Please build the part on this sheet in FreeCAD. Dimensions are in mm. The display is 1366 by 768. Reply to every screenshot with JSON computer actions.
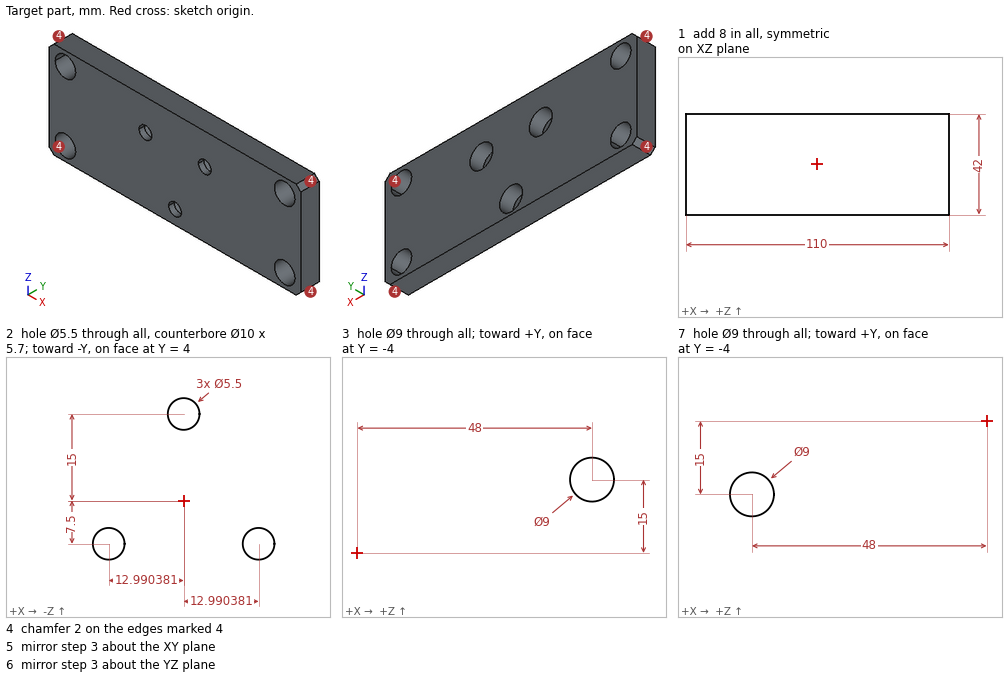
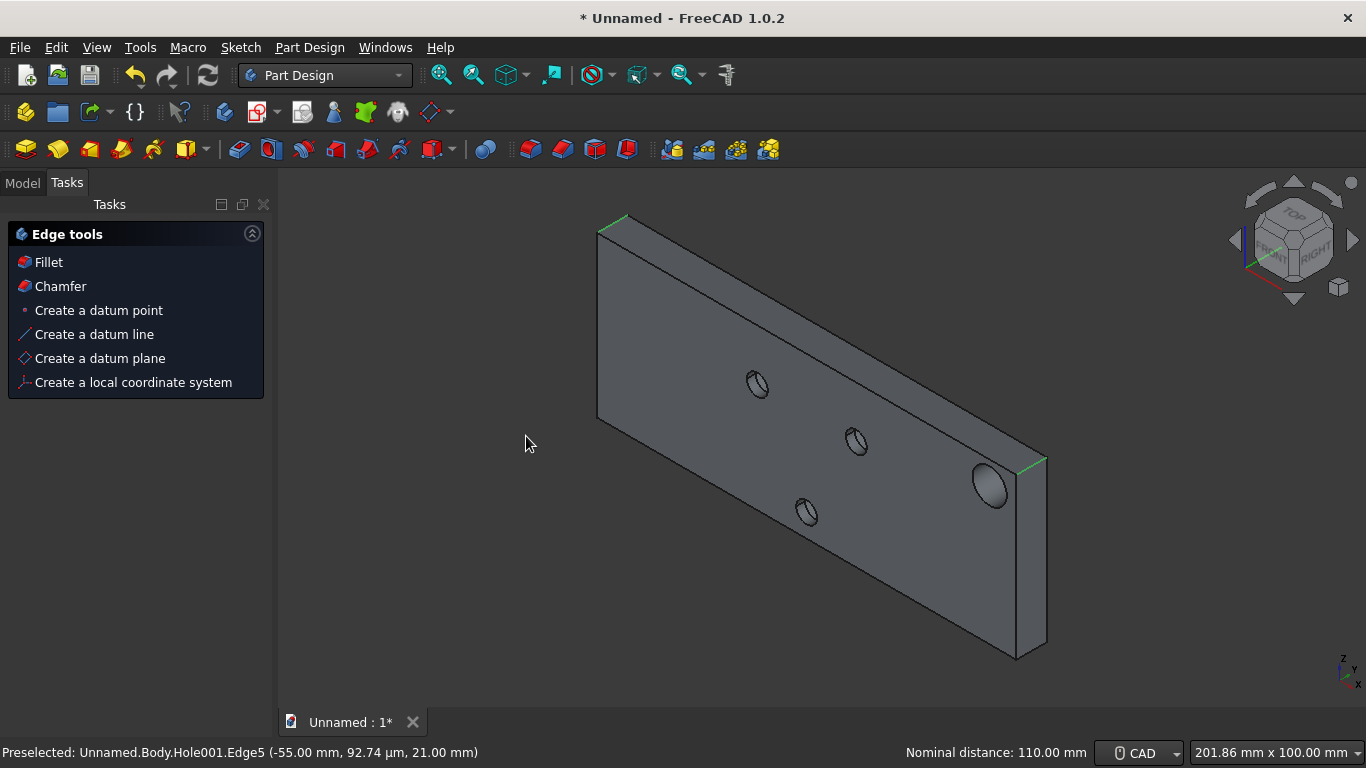
{"action": "key", "text": "1"}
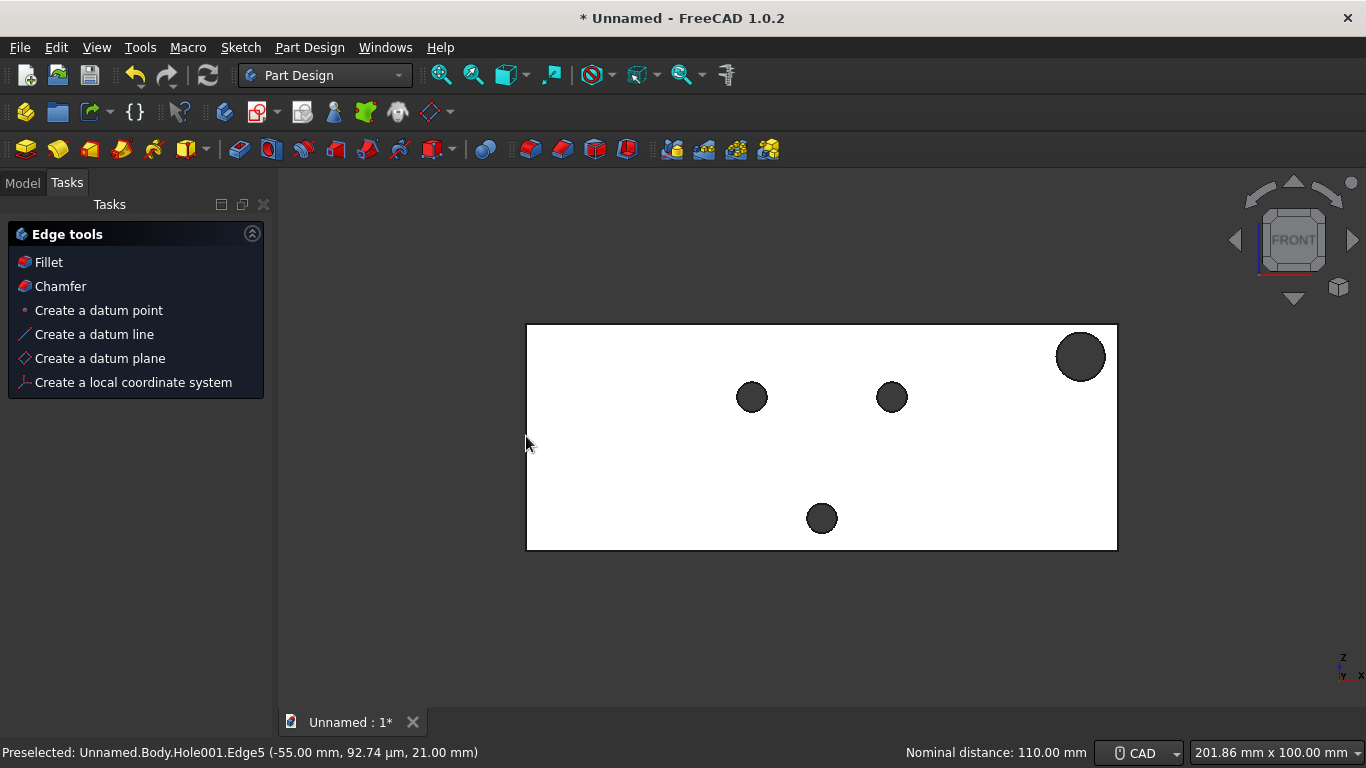
{"action": "key", "text": "3"}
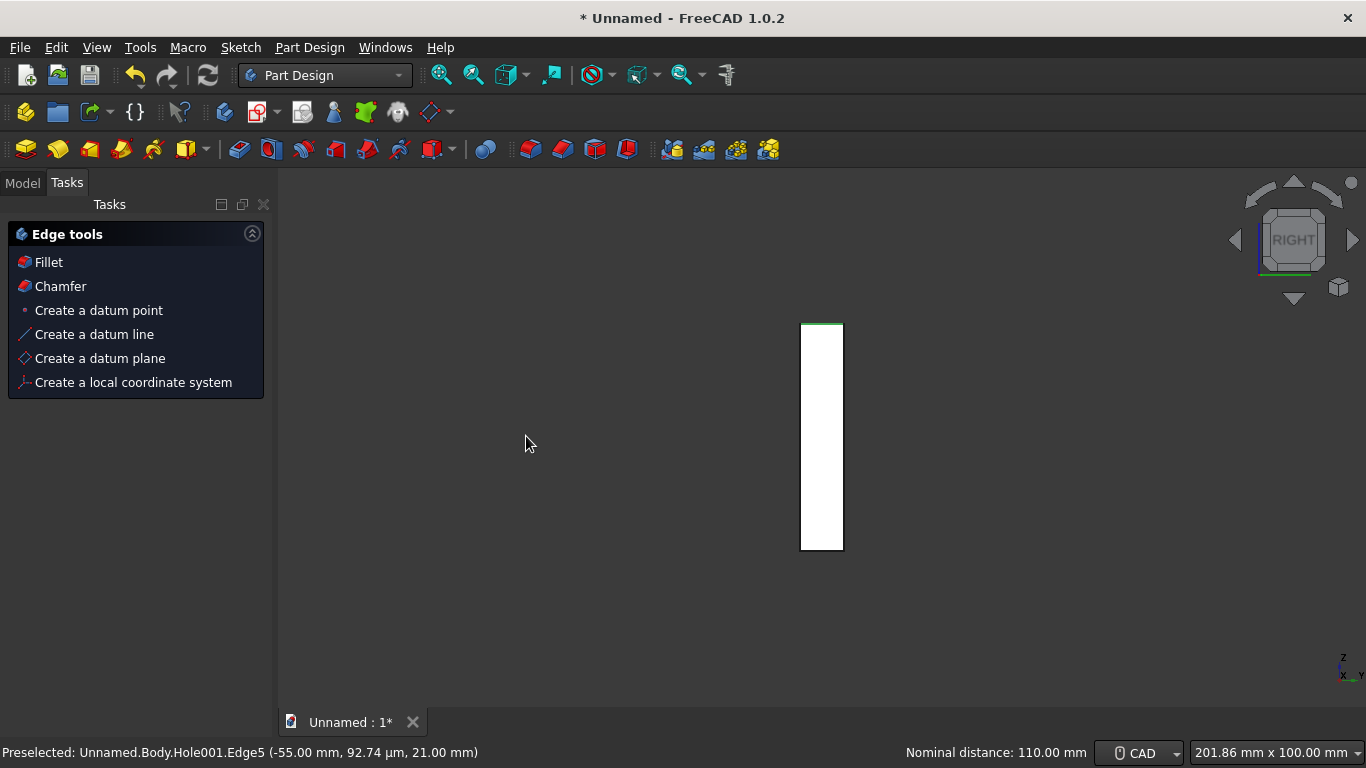
{"action": "left_click", "coordinate": [442, 76]}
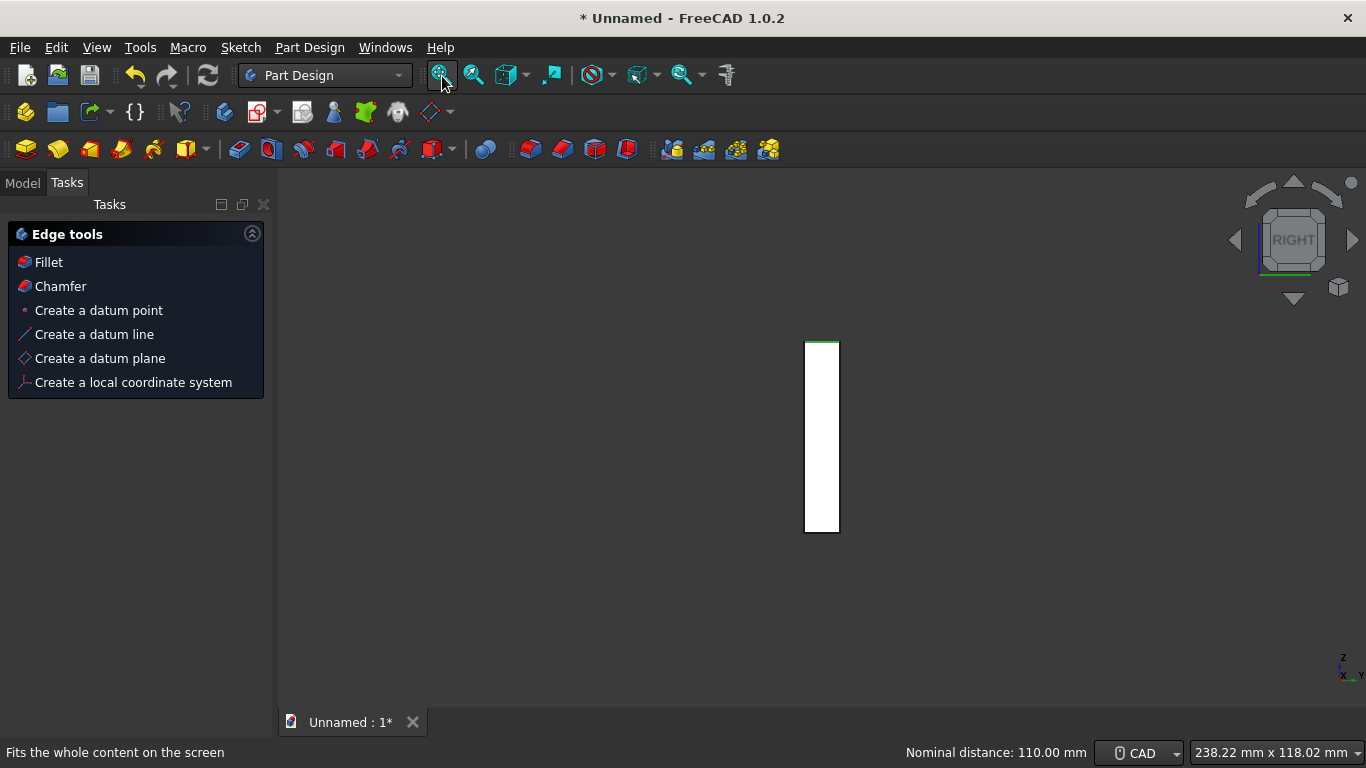
{"action": "left_click", "coordinate": [822, 532], "text": "ctrl"}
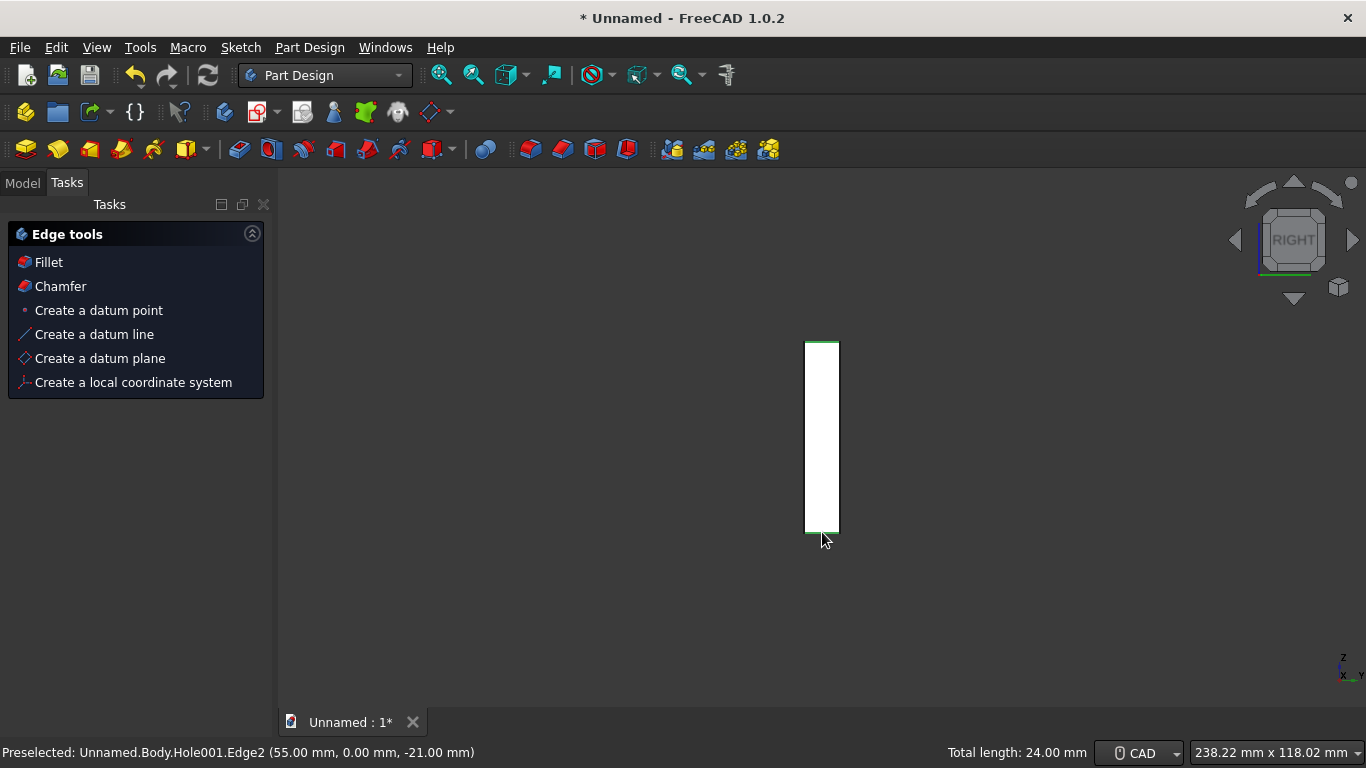
{"action": "key", "text": "5"}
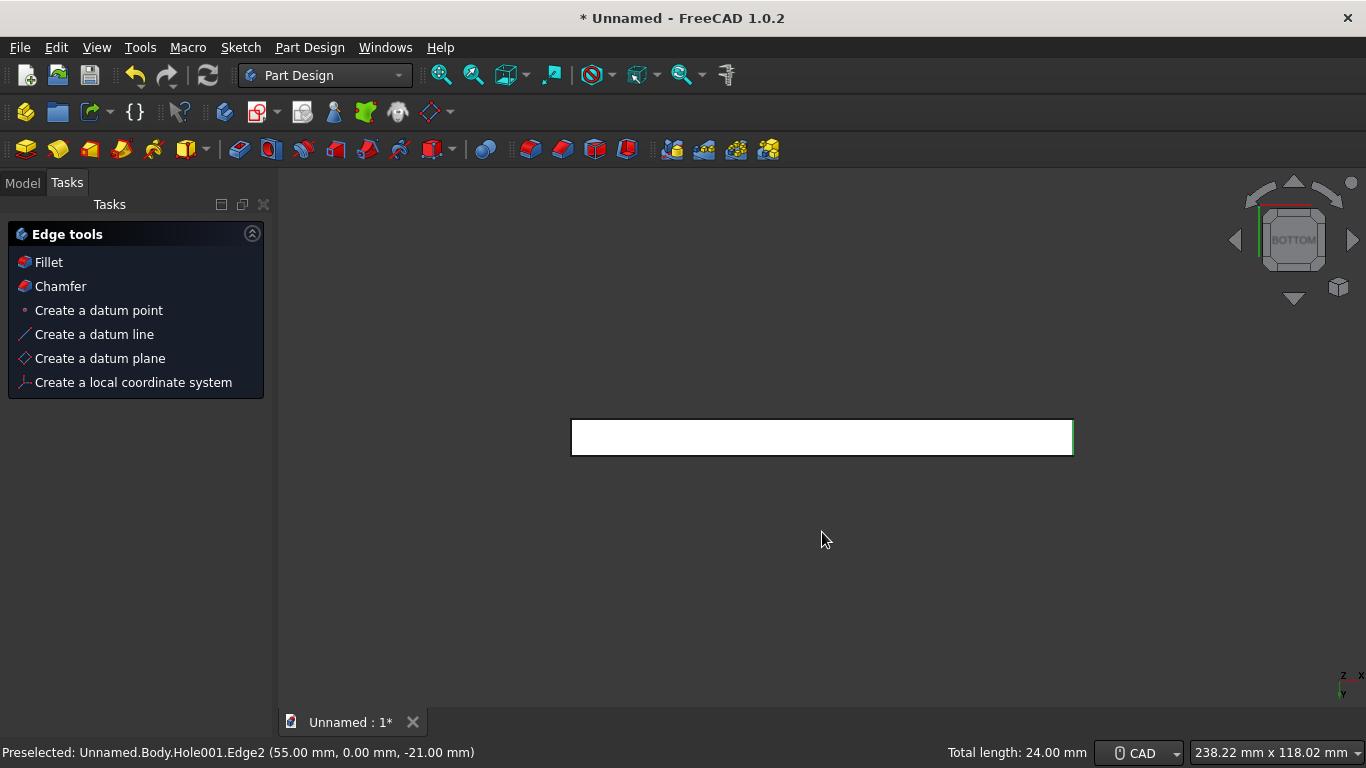
{"action": "left_click", "coordinate": [571, 436], "text": "ctrl"}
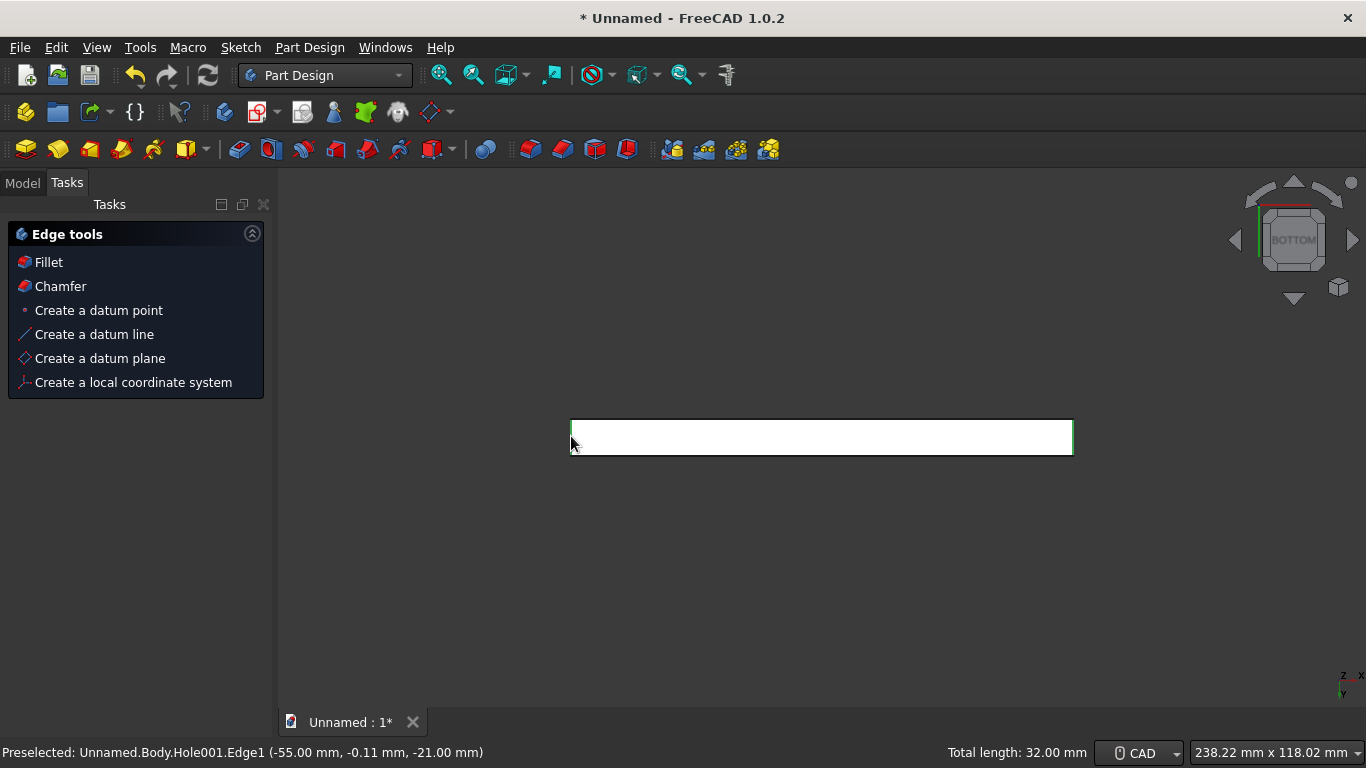
{"action": "left_click", "coordinate": [564, 150]}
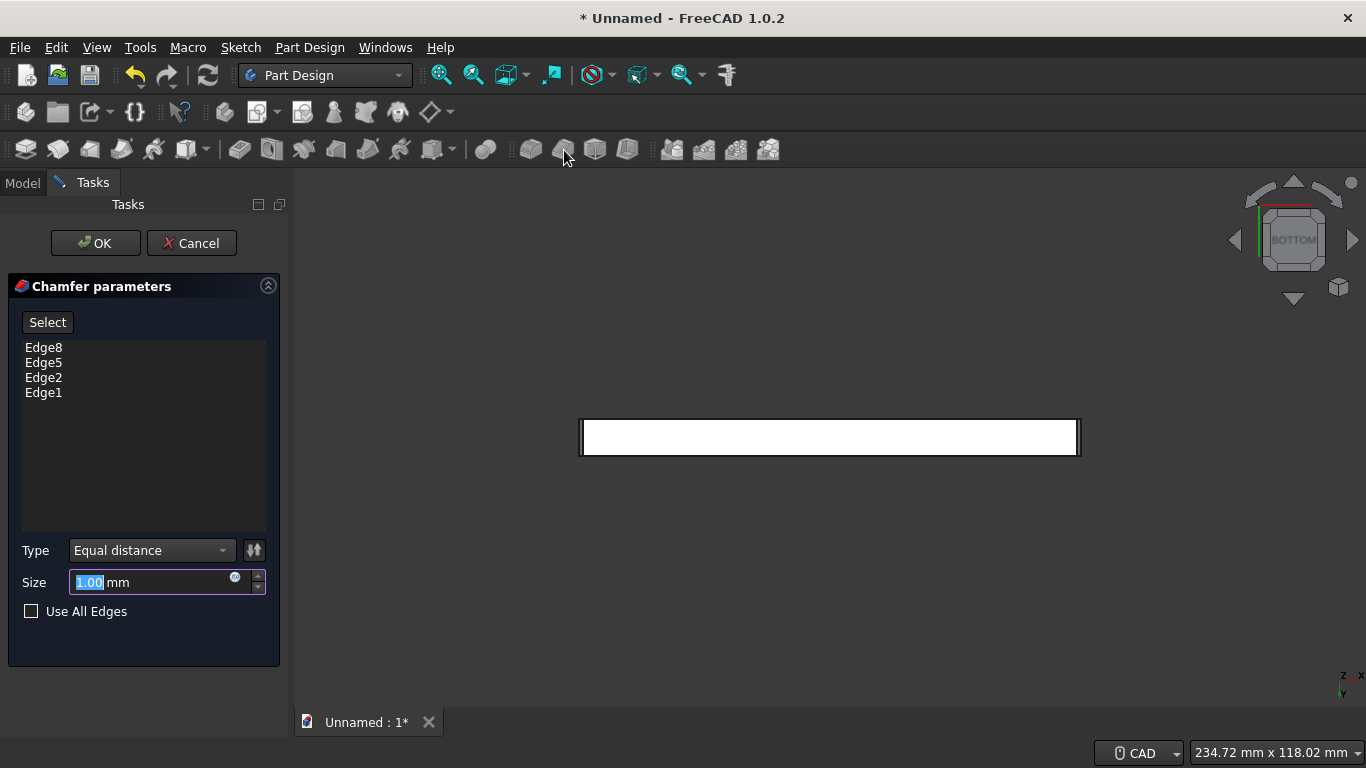
{"action": "type", "text": "2"}
{"action": "key", "text": "Tab"}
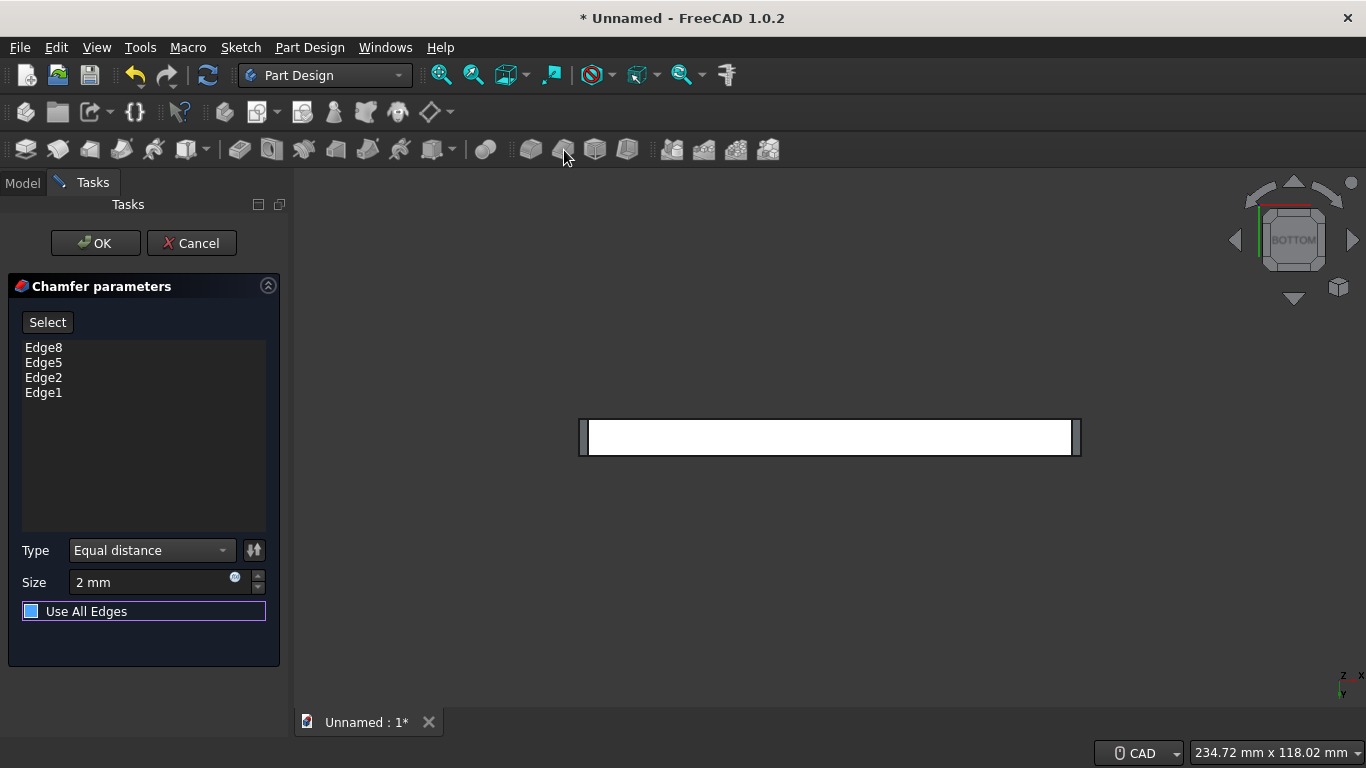
{"action": "left_click", "coordinate": [96, 243]}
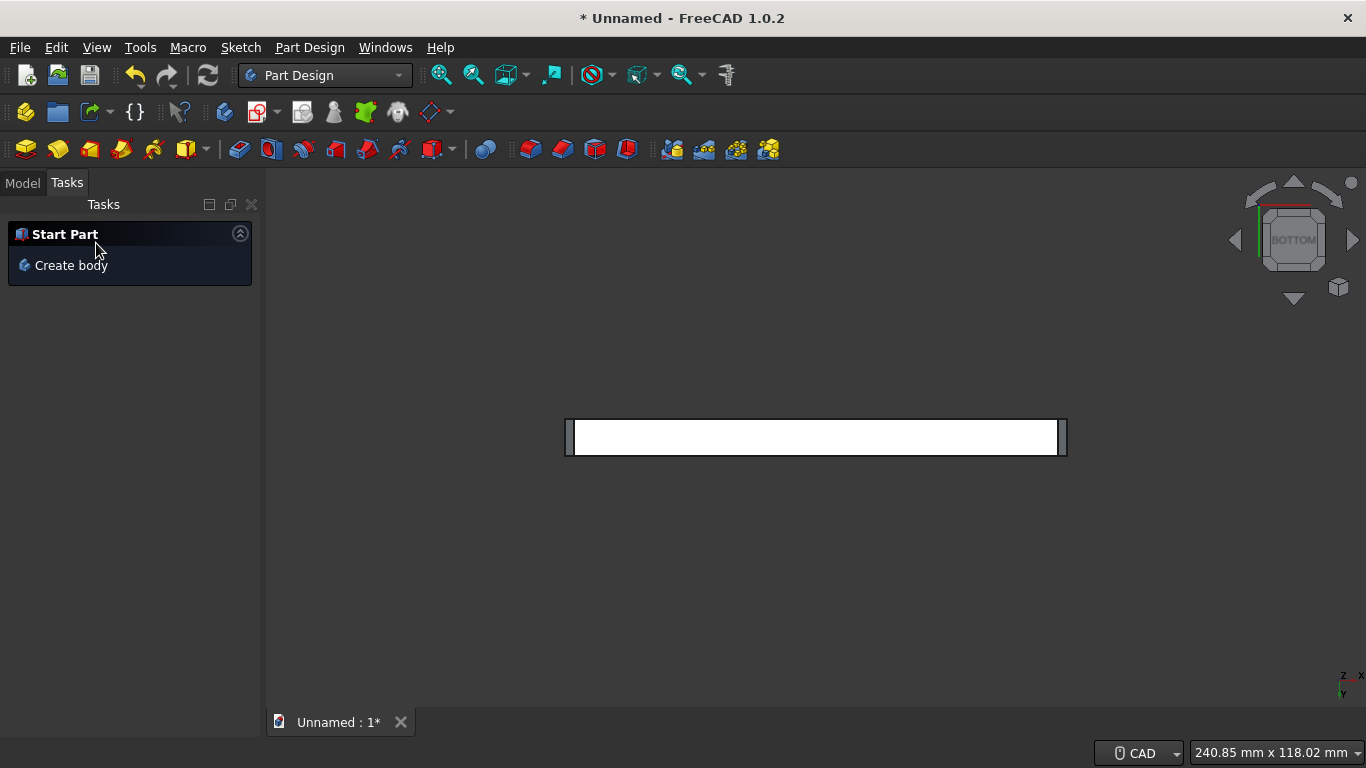
{"action": "left_click", "coordinate": [23, 182]}